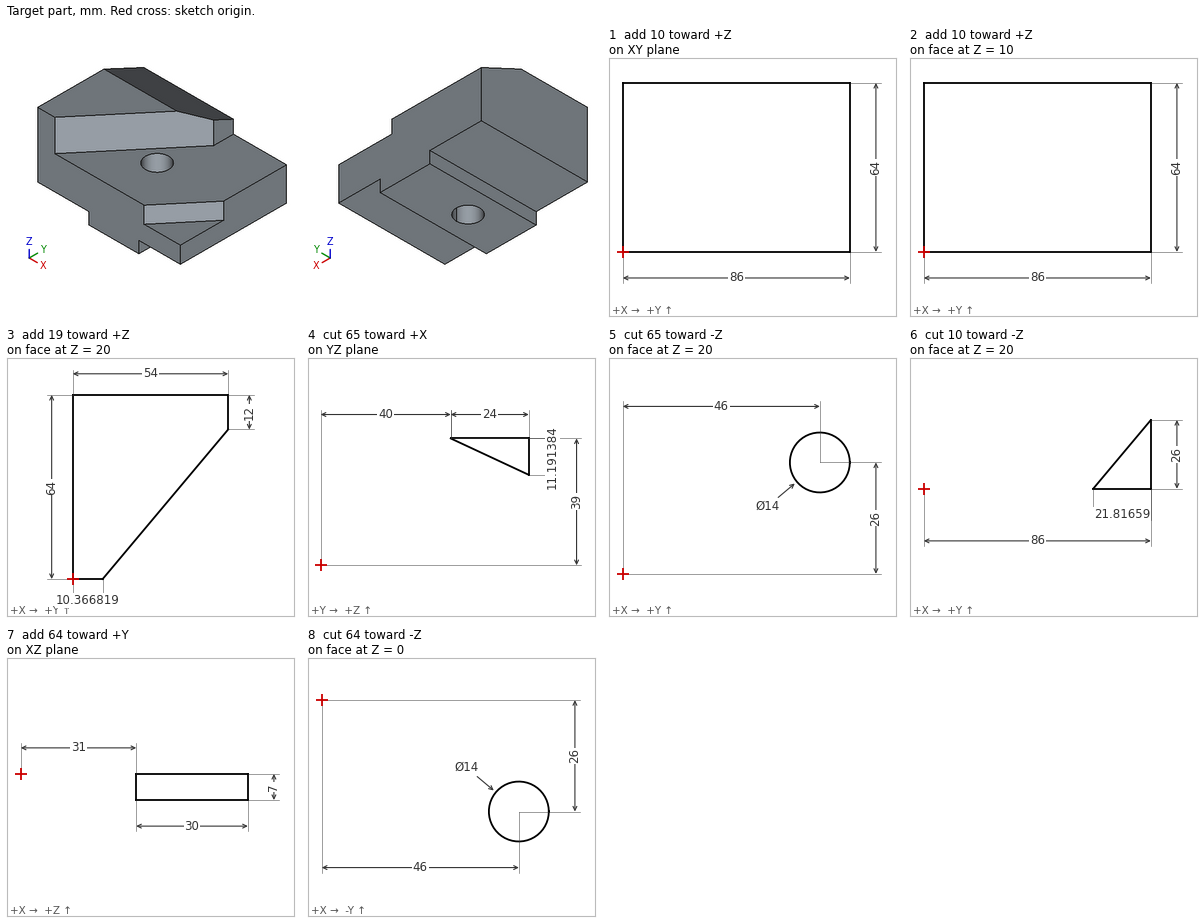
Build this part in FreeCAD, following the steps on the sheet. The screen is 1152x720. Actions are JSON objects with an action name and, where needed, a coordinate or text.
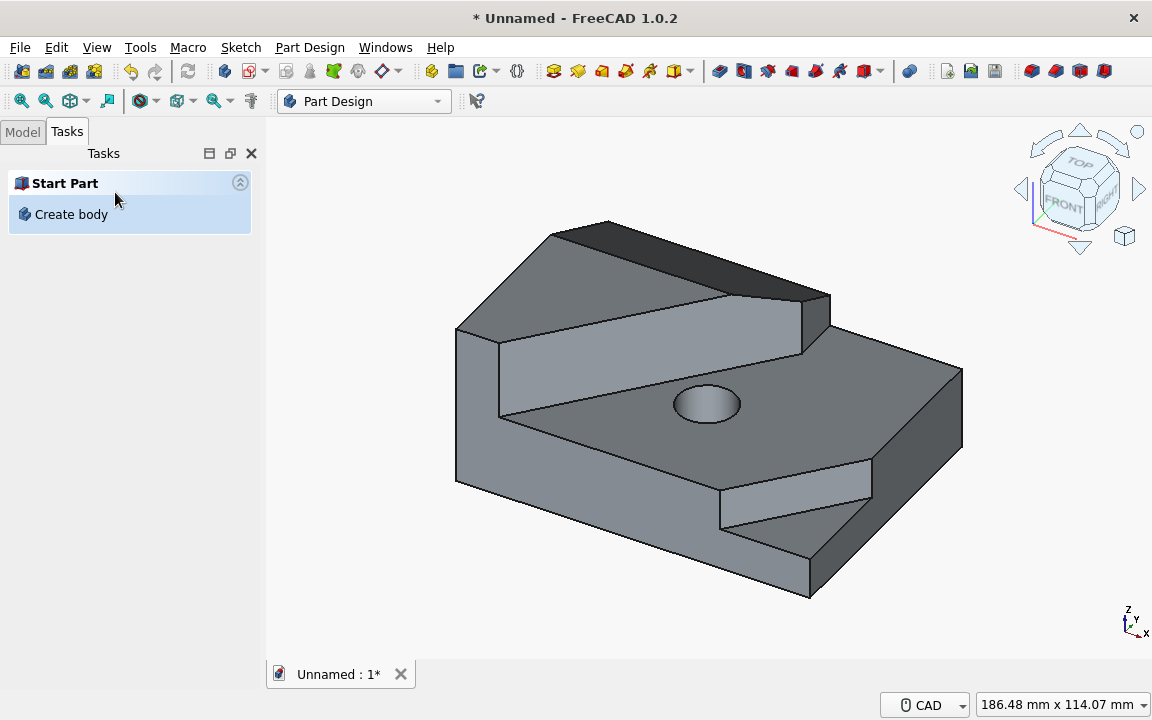
{"action": "left_click", "coordinate": [250, 72]}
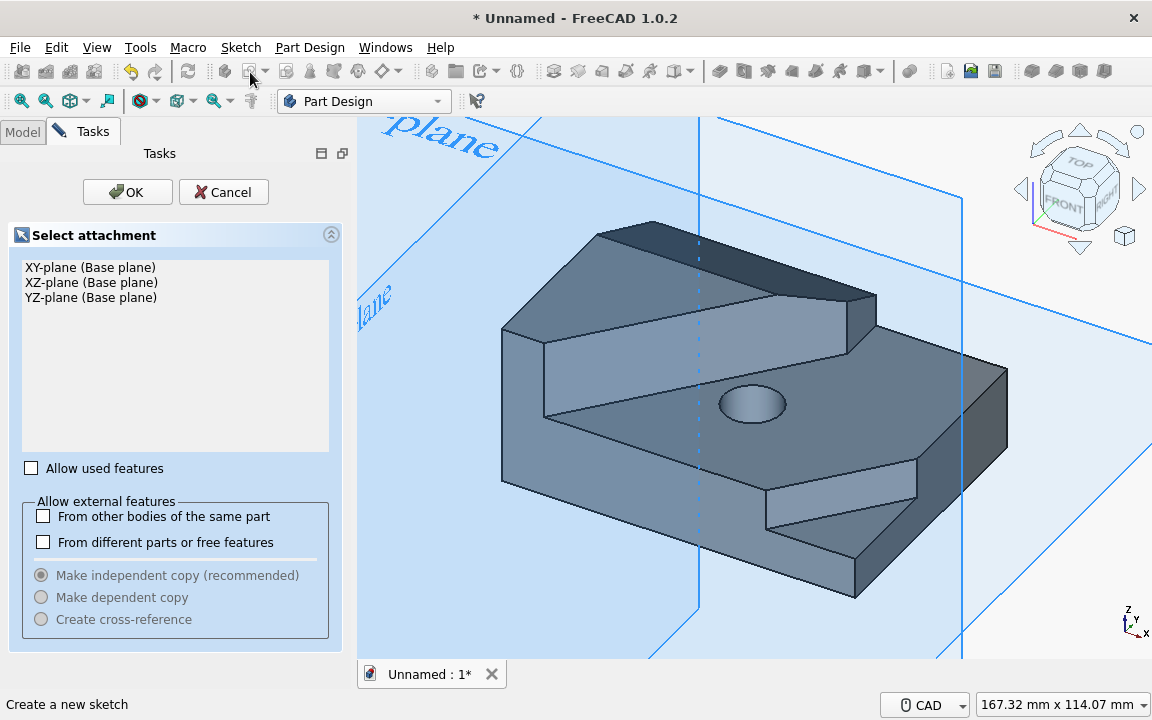
{"action": "left_click", "coordinate": [82, 282]}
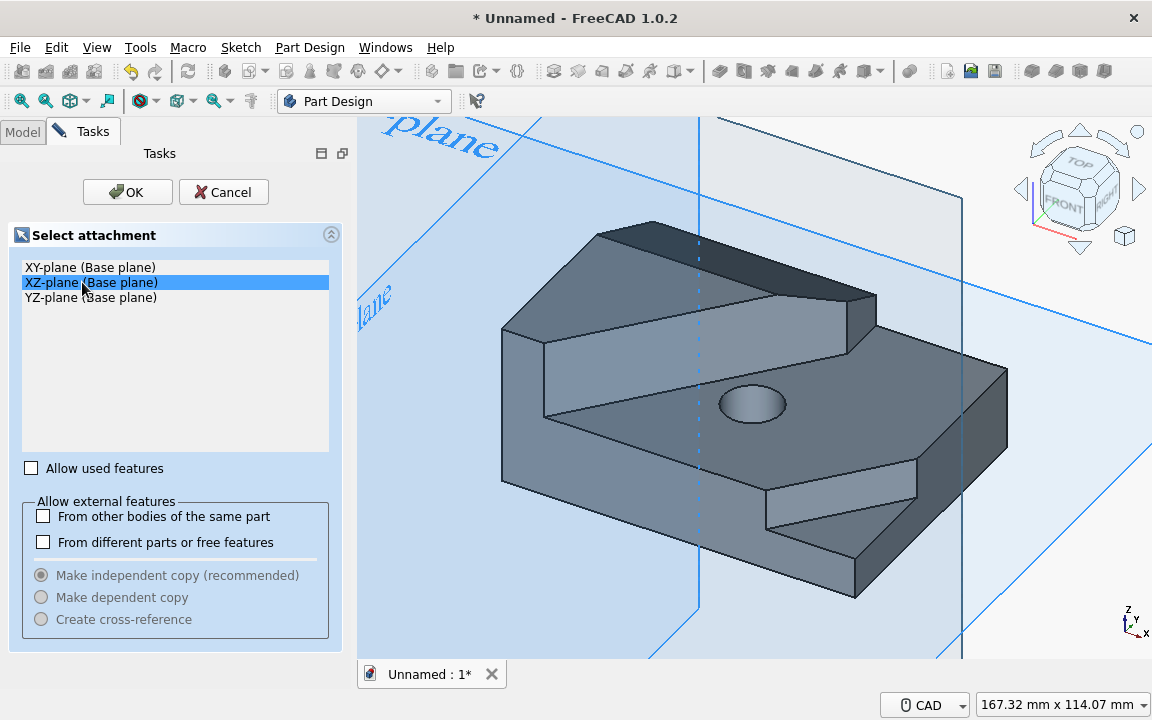
{"action": "left_click", "coordinate": [128, 192]}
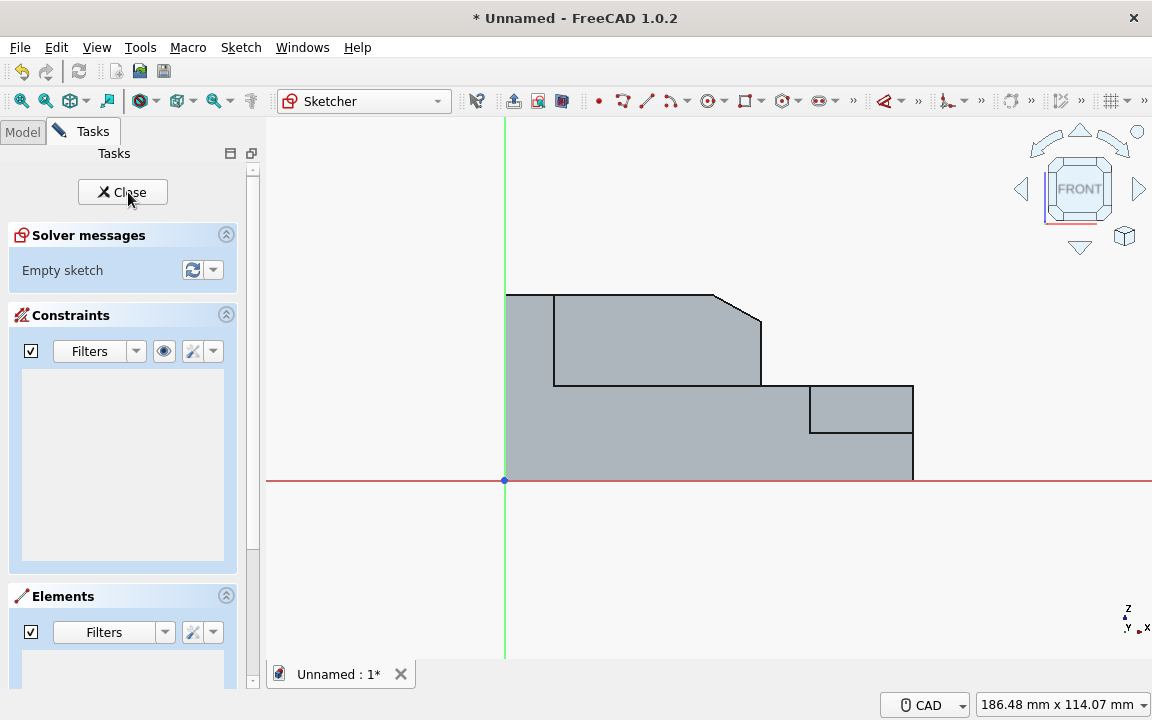
{"action": "scroll", "coordinate": [661, 630], "scroll_direction": "up", "scroll_amount": 3}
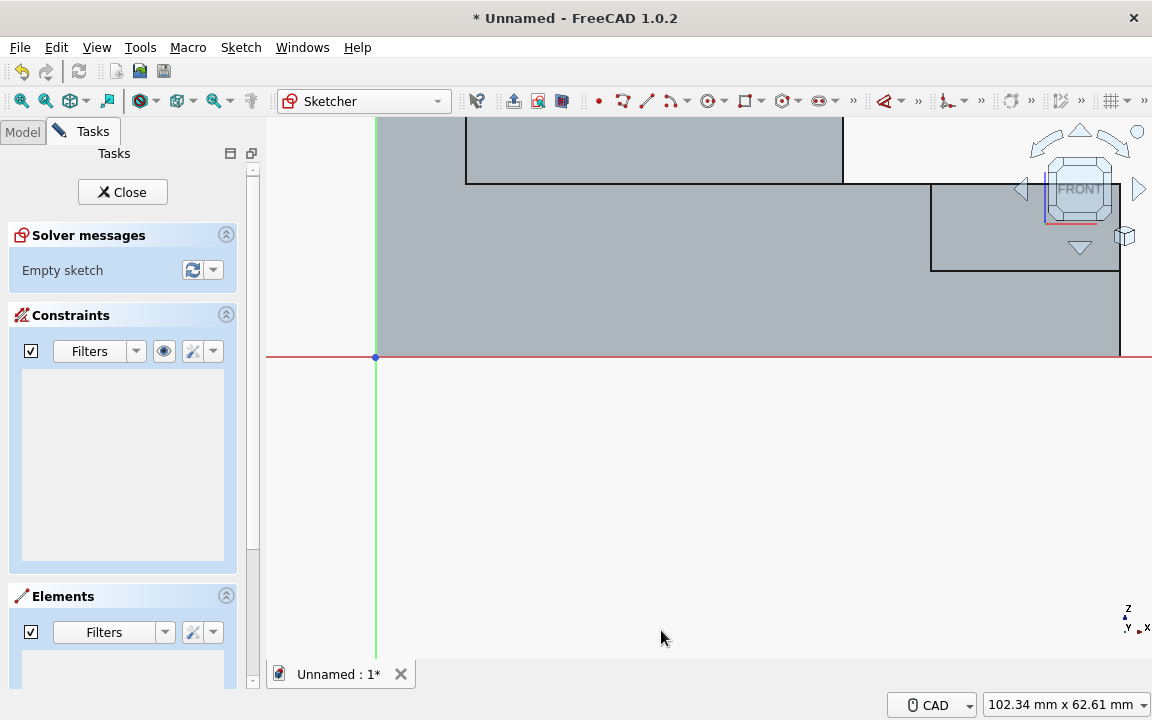
{"action": "left_click", "coordinate": [746, 102]}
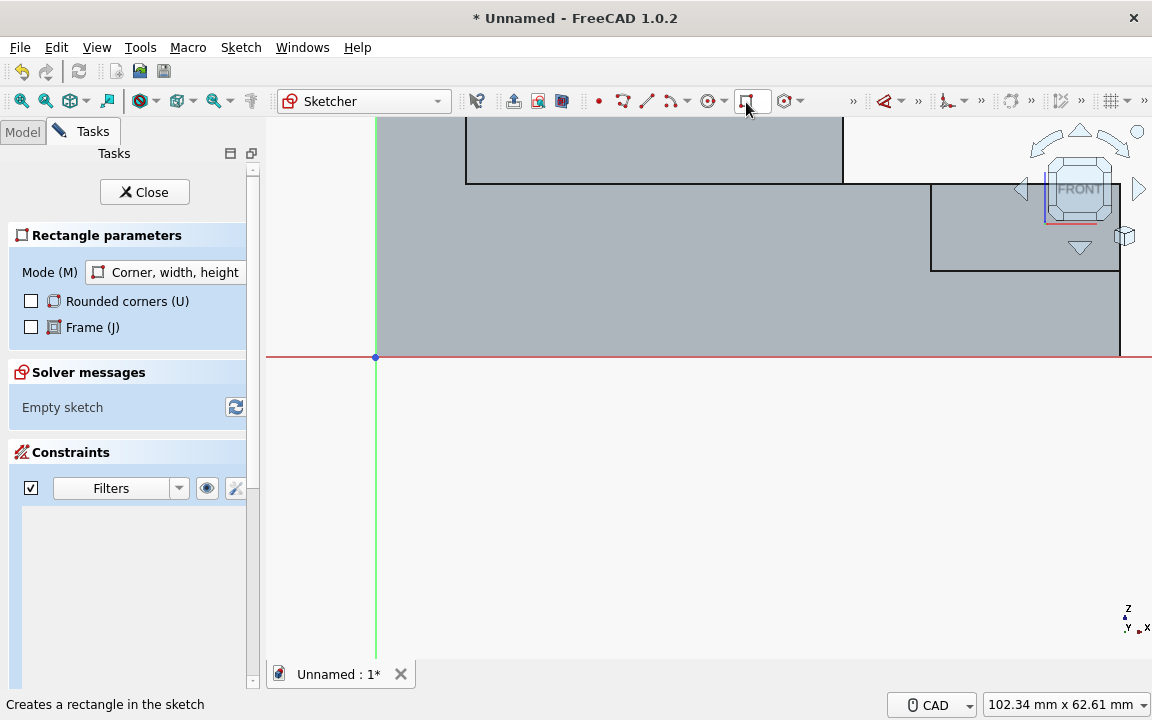
{"action": "left_click", "coordinate": [644, 357]}
{"action": "mouse_move", "coordinate": [904, 418]}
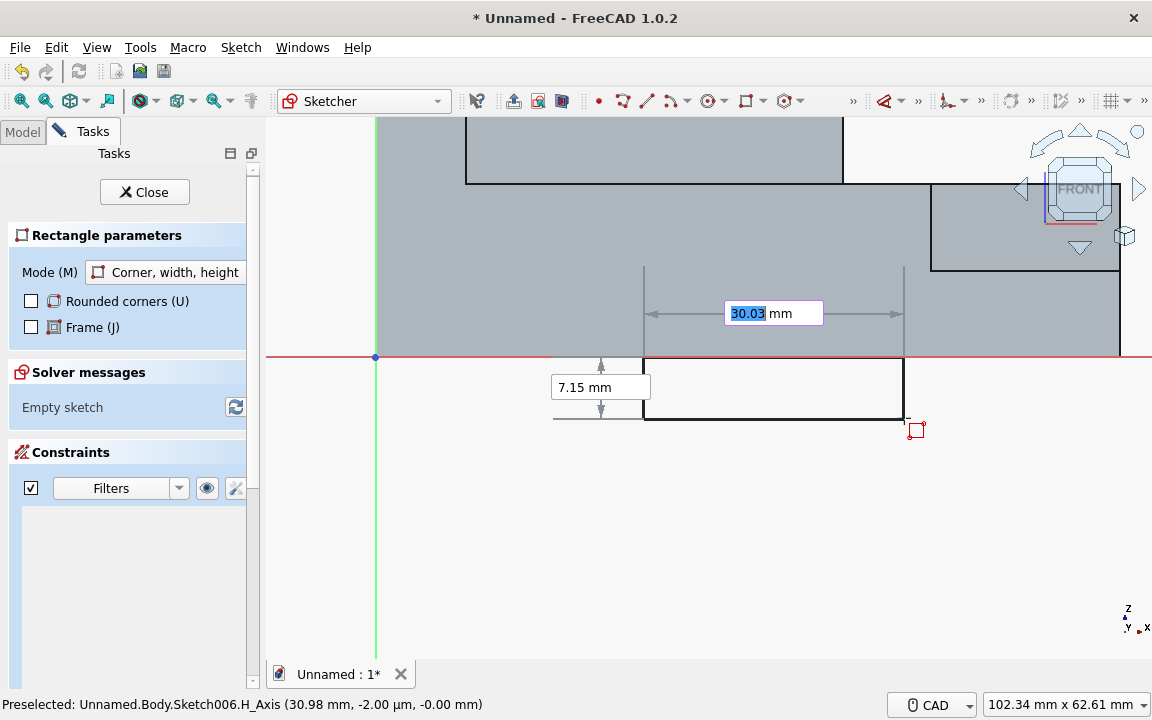
{"action": "type", "text": "30"}
{"action": "key", "text": "Tab"}
{"action": "type", "text": "7"}
{"action": "key", "text": "Return"}
{"action": "key", "text": "Escape"}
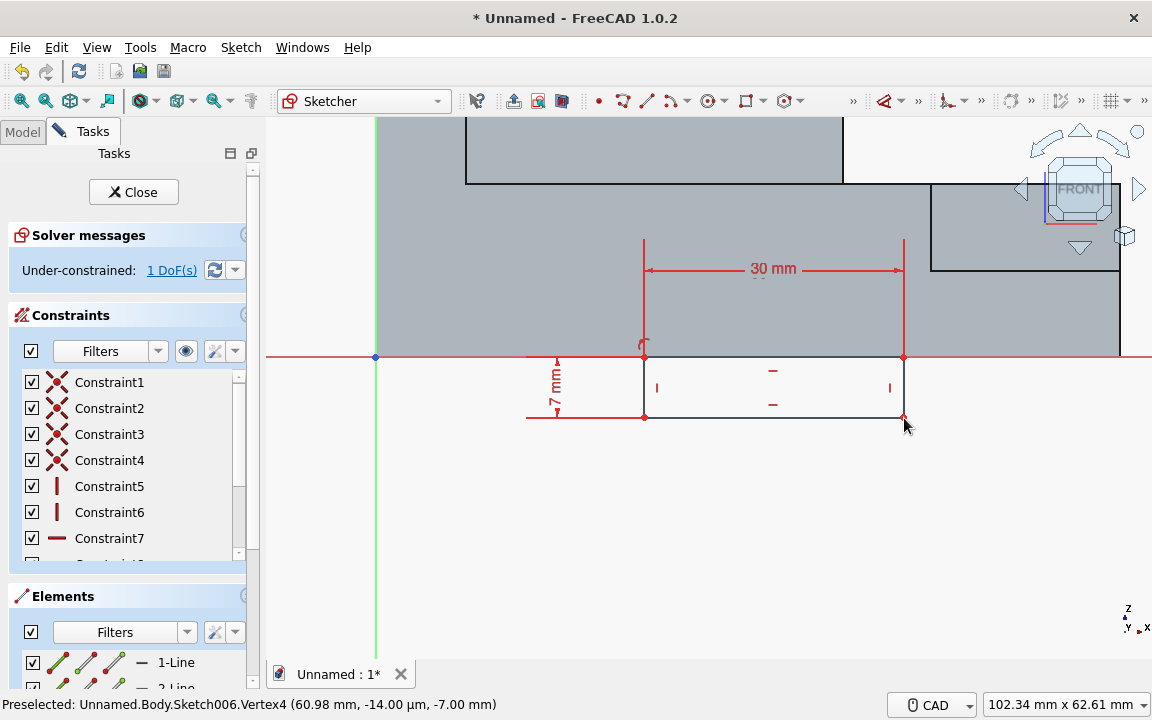
{"action": "left_click", "coordinate": [884, 102]}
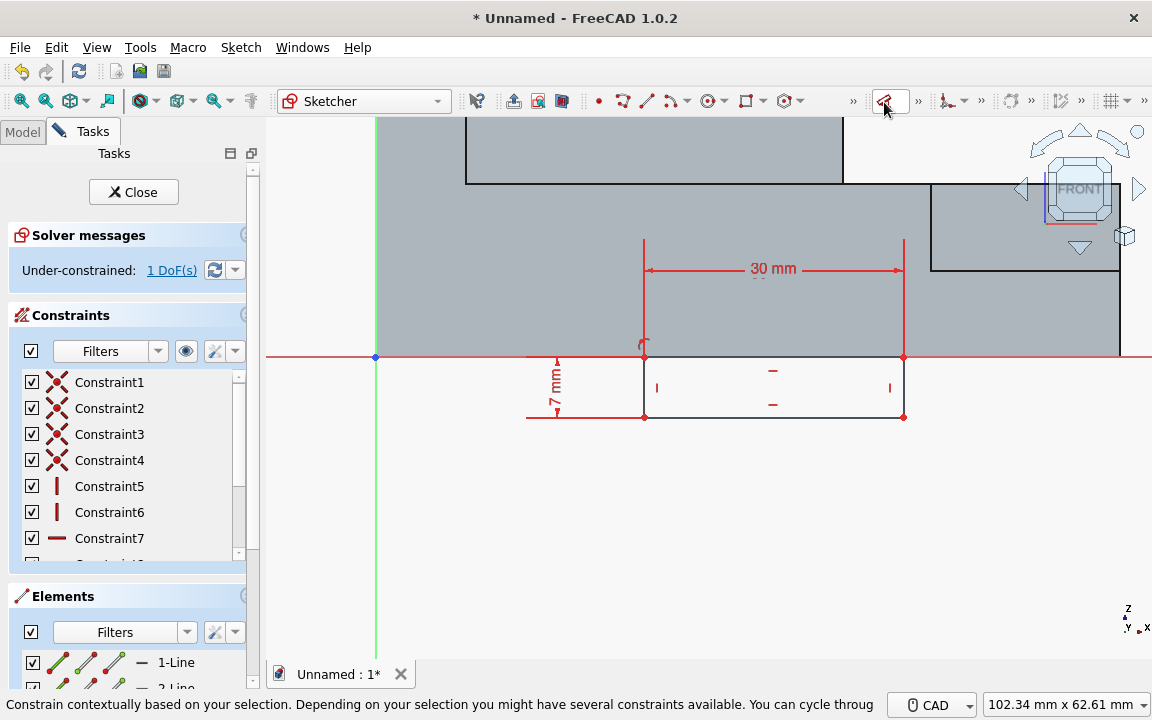
{"action": "left_click", "coordinate": [644, 357]}
{"action": "left_click", "coordinate": [510, 323]}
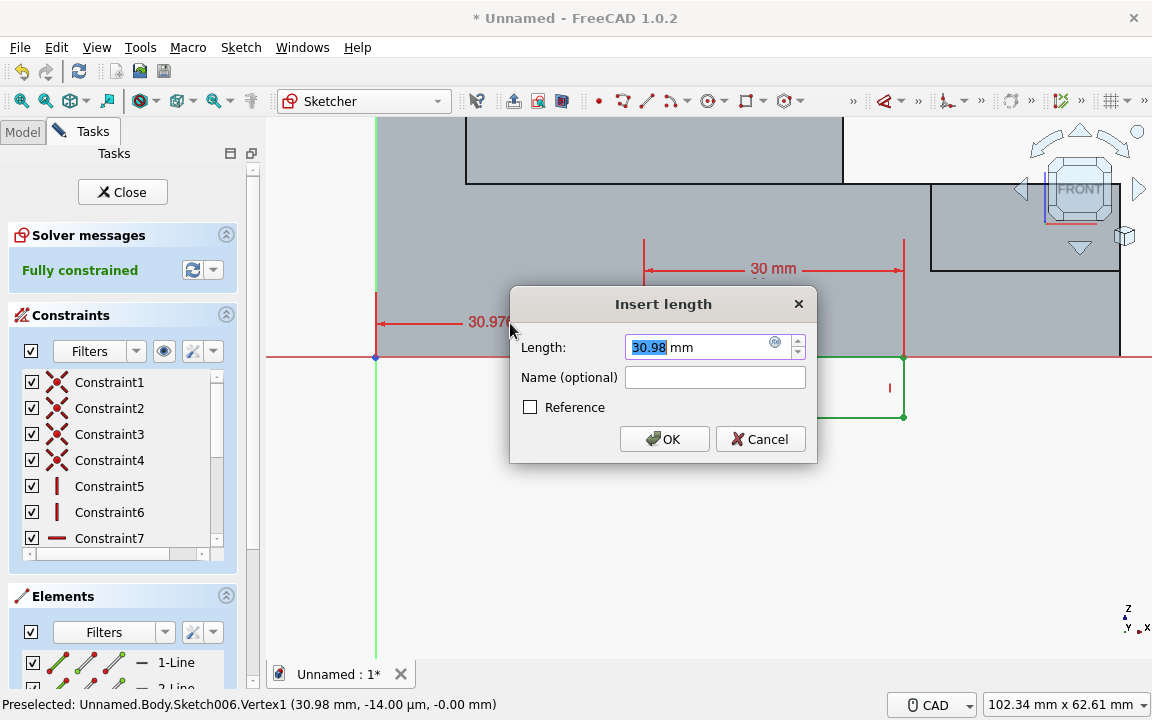
{"action": "type", "text": "31"}
{"action": "key", "text": "Return"}
{"action": "key", "text": "Escape"}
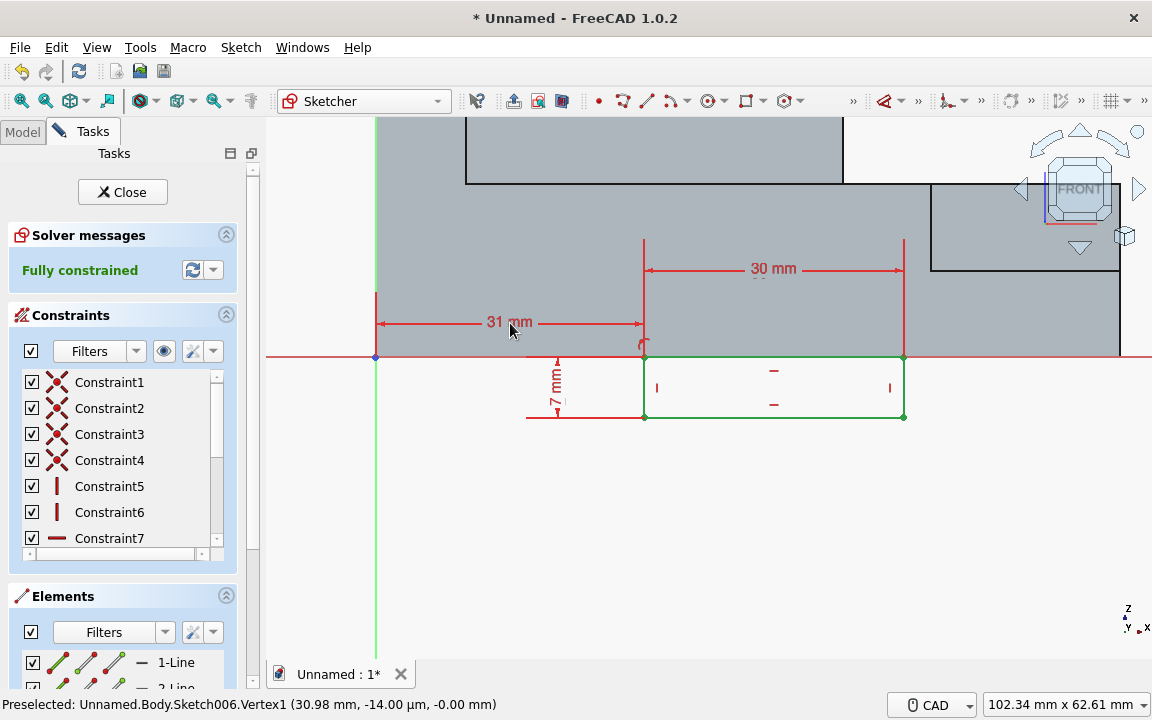
{"action": "left_click", "coordinate": [123, 192]}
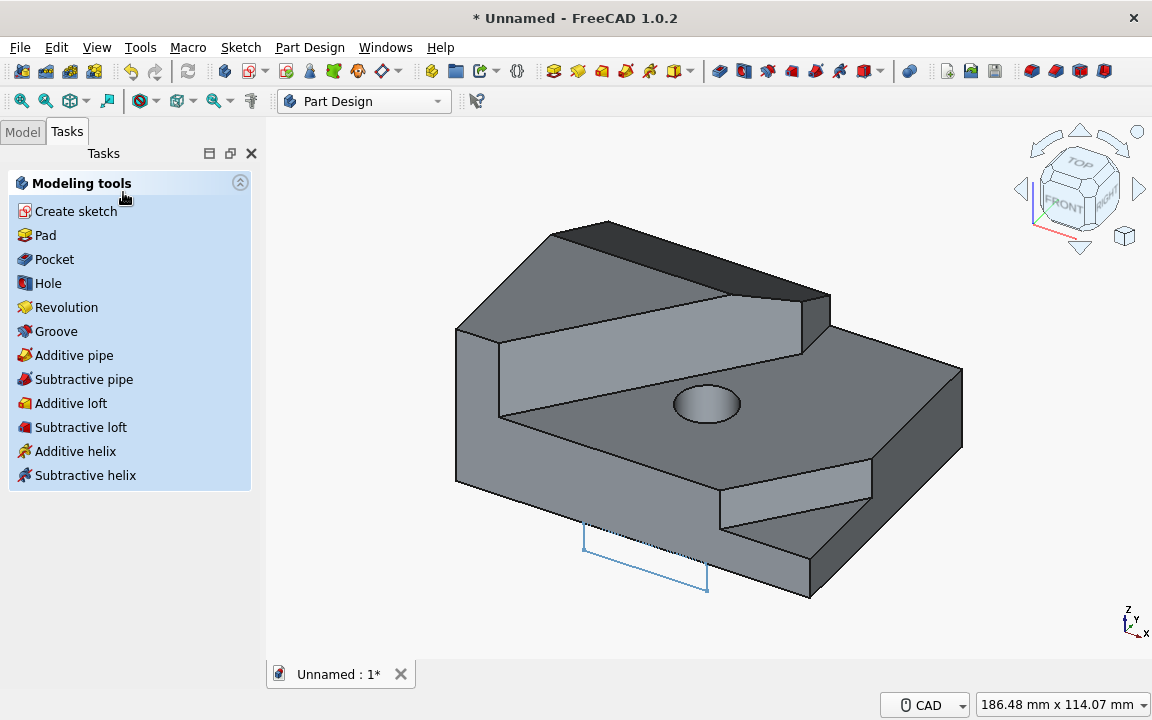
{"action": "left_click", "coordinate": [554, 72]}